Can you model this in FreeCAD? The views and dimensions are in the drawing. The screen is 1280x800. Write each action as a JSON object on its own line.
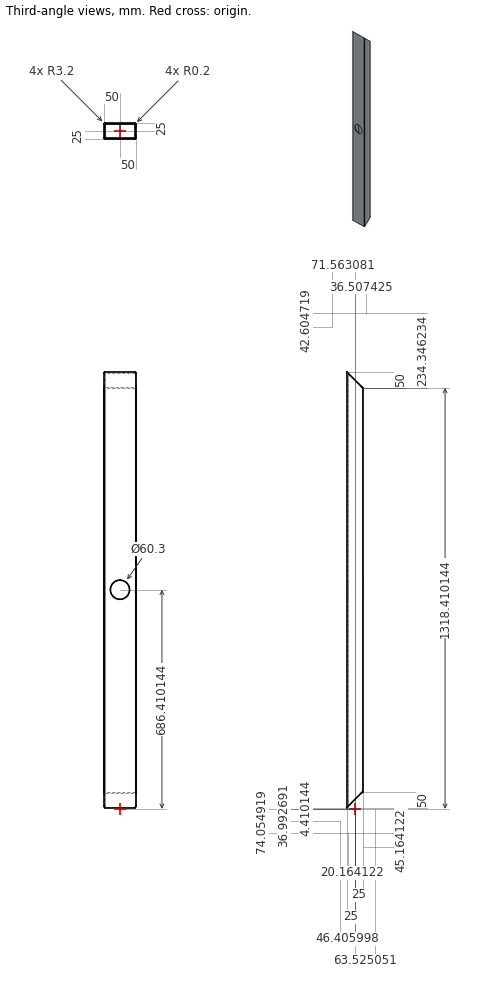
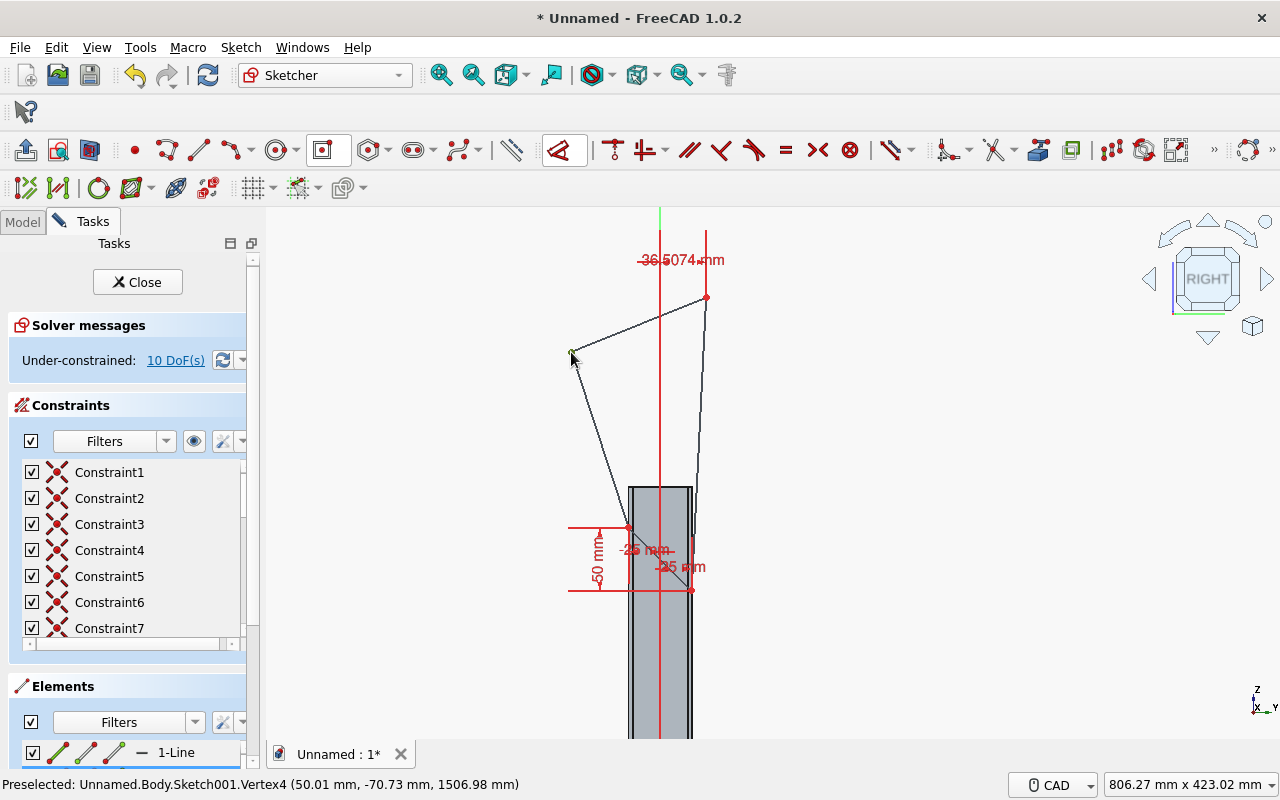
{"action": "key", "text": "l"}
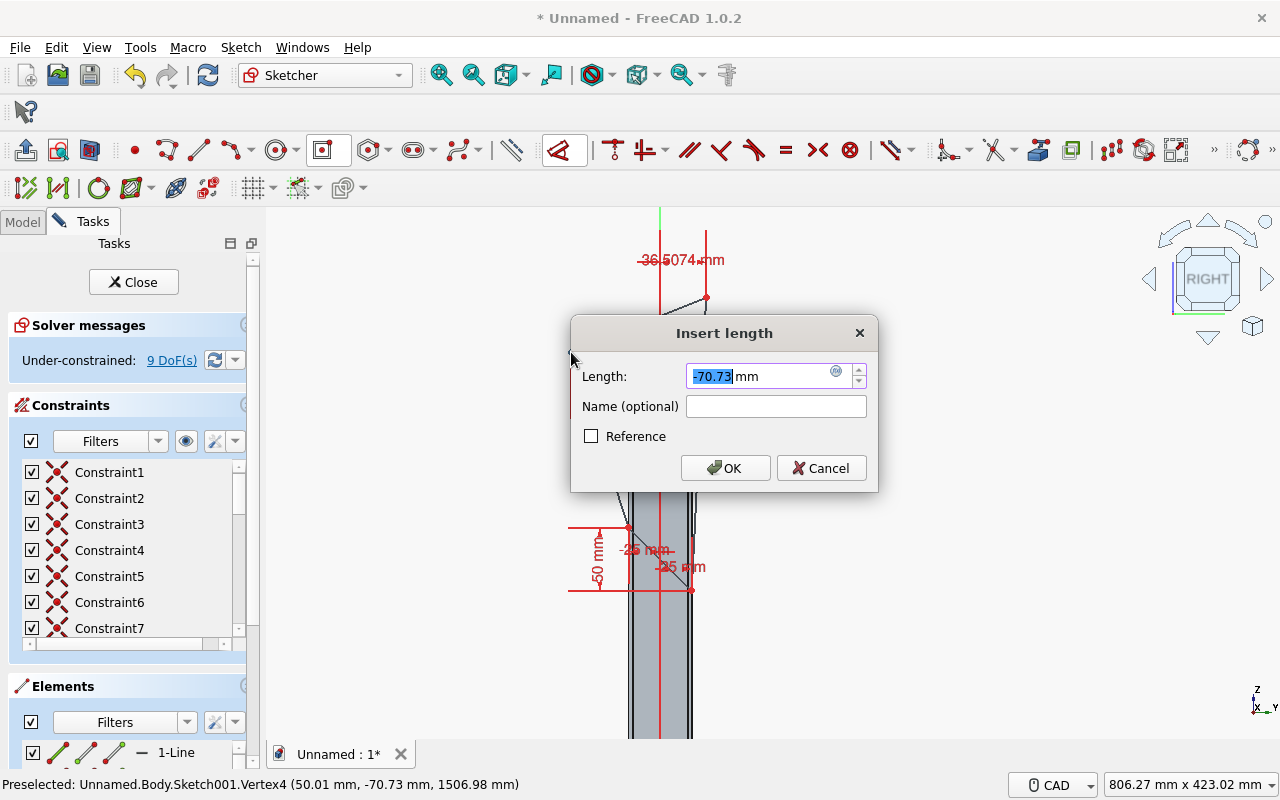
{"action": "type", "text": "-71.563081"}
{"action": "key", "text": "Return"}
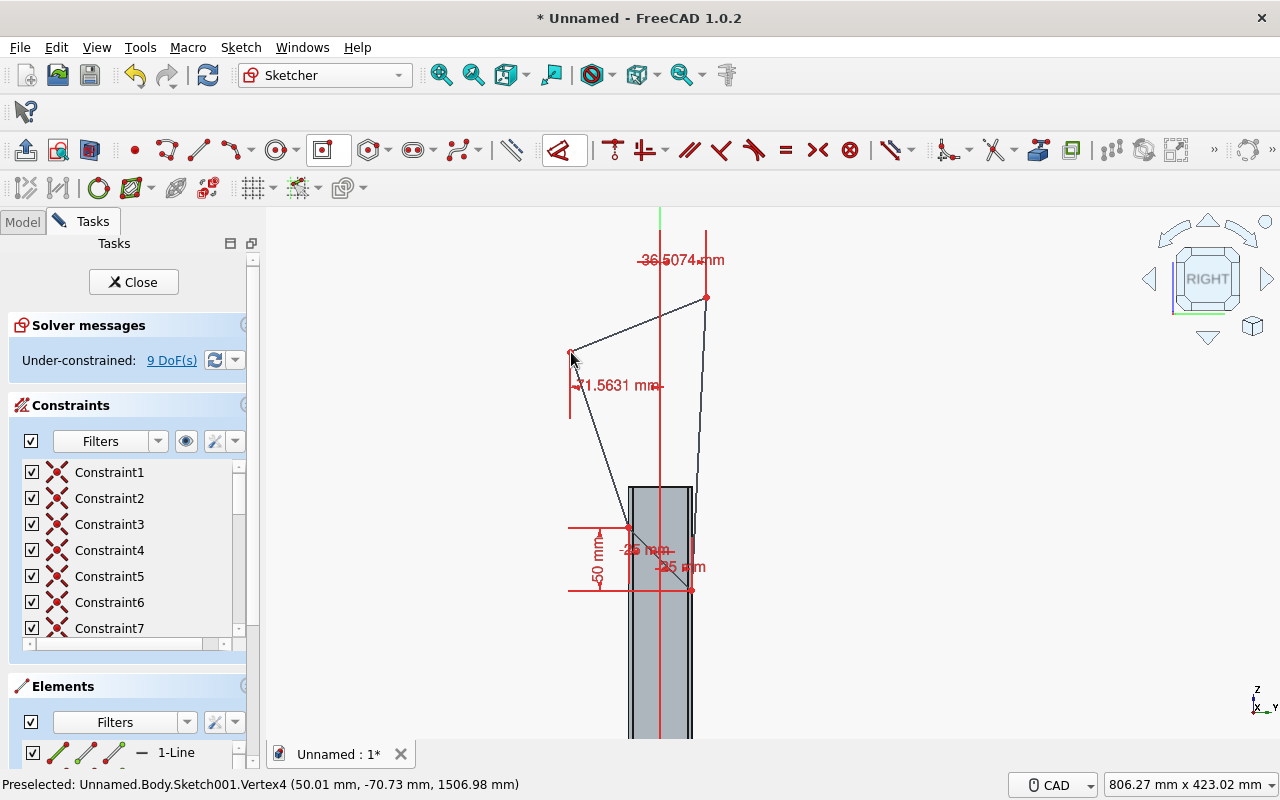
{"action": "scroll", "coordinate": [714, 300], "scroll_direction": "down", "scroll_amount": 9}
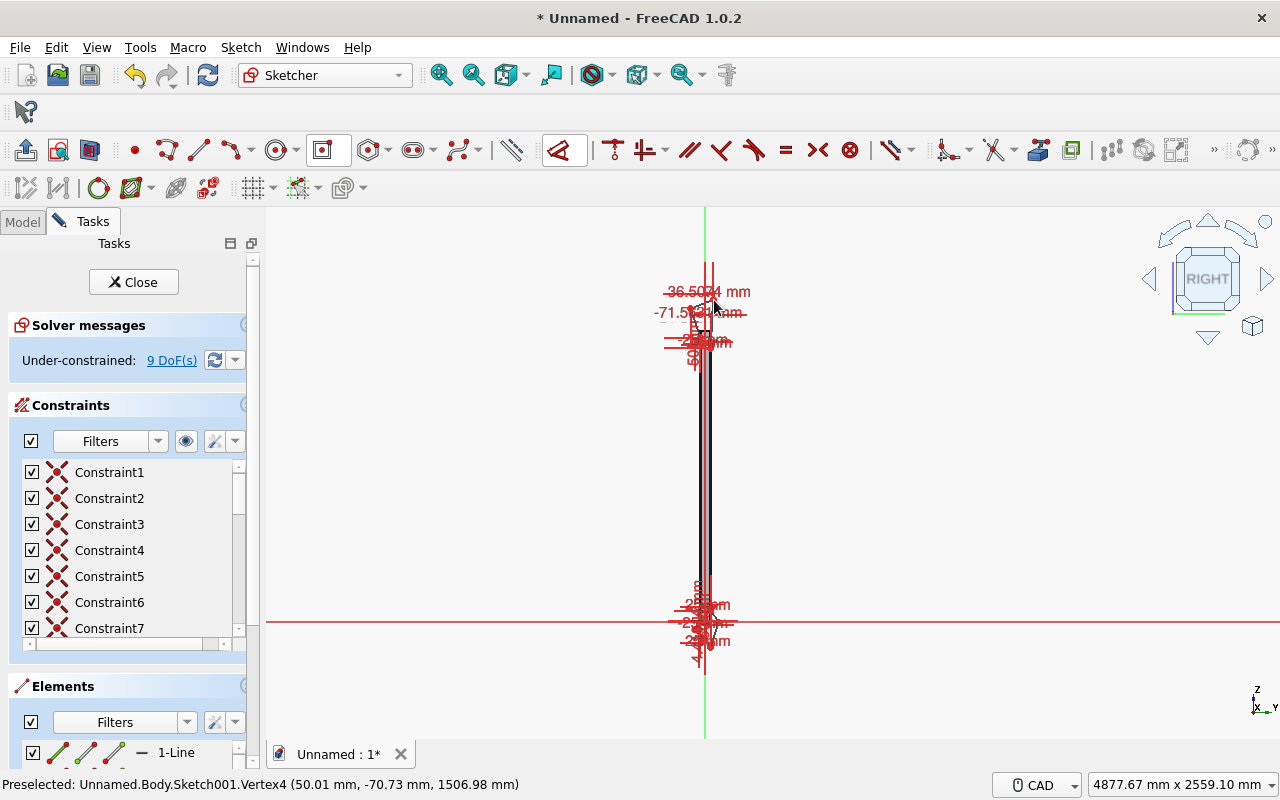
{"action": "scroll", "coordinate": [696, 630], "scroll_direction": "up", "scroll_amount": 8}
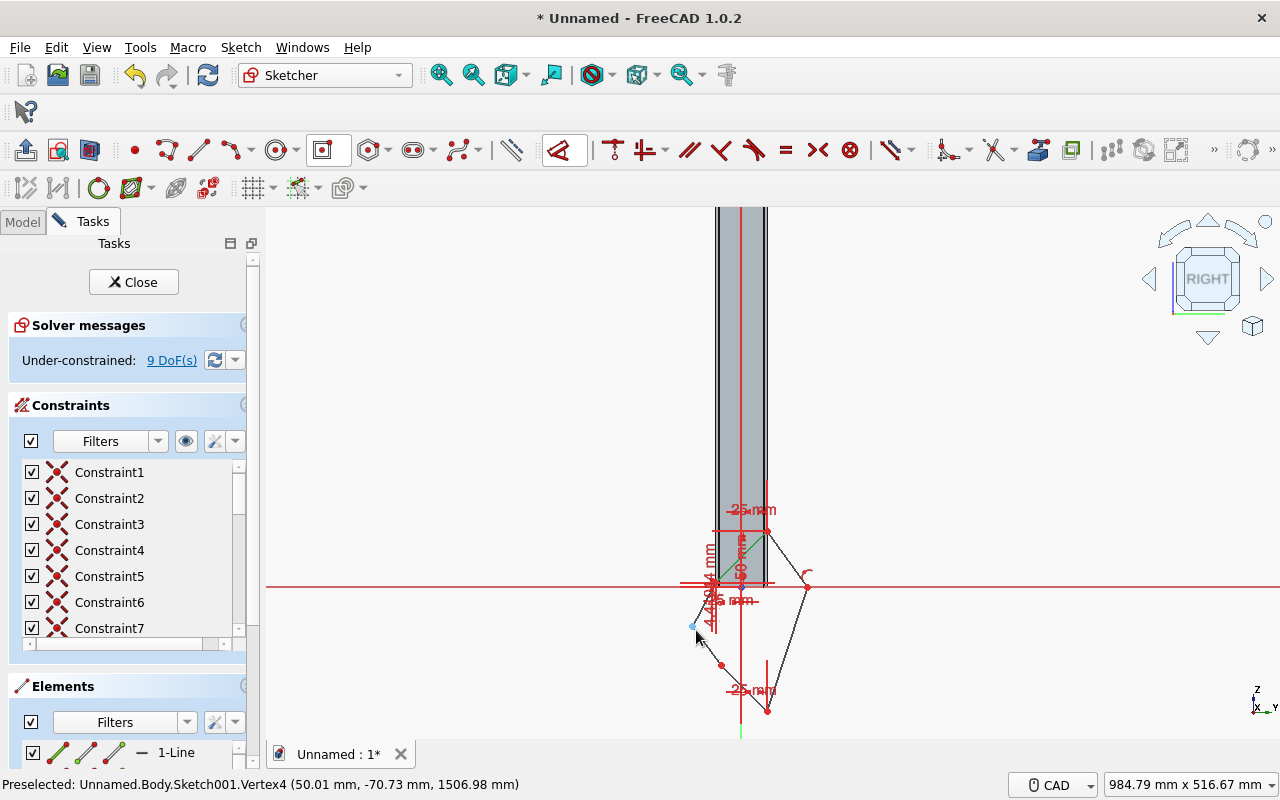
{"action": "left_click", "coordinate": [693, 627]}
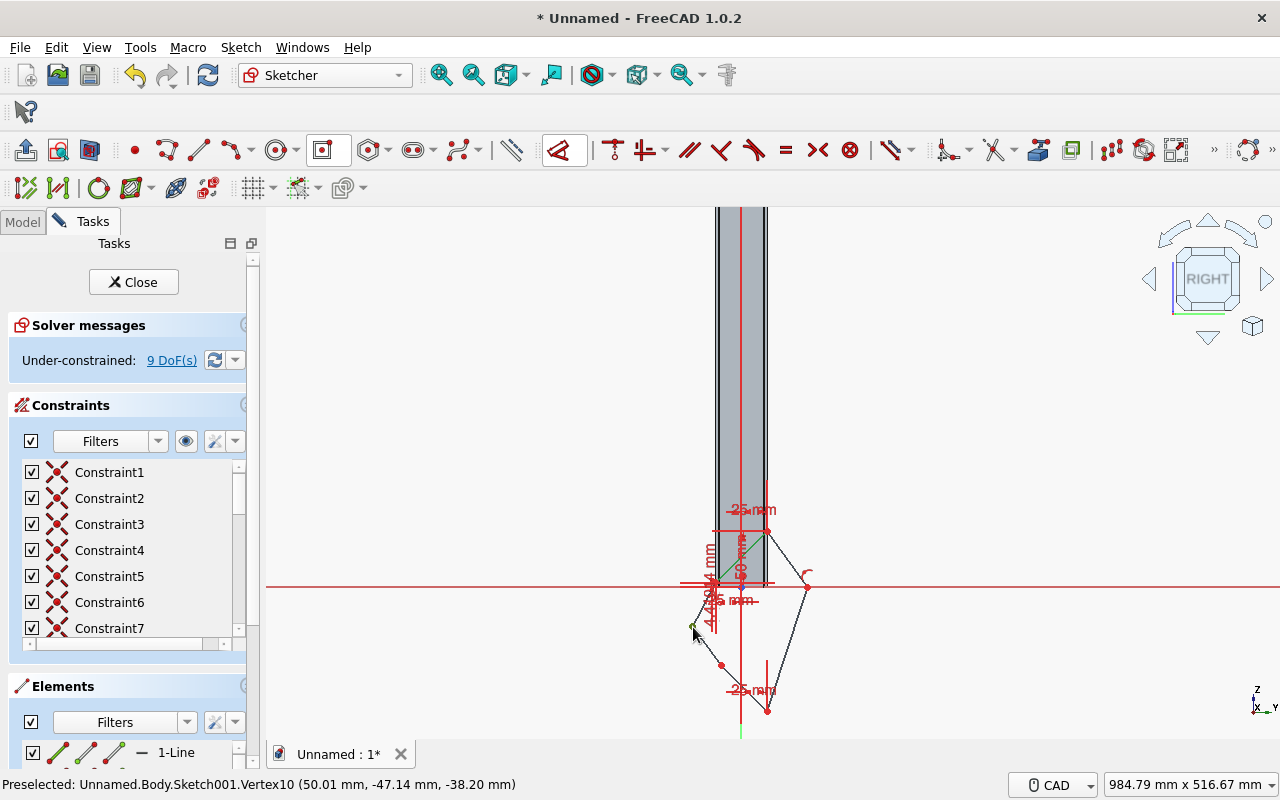
{"action": "key", "text": "l"}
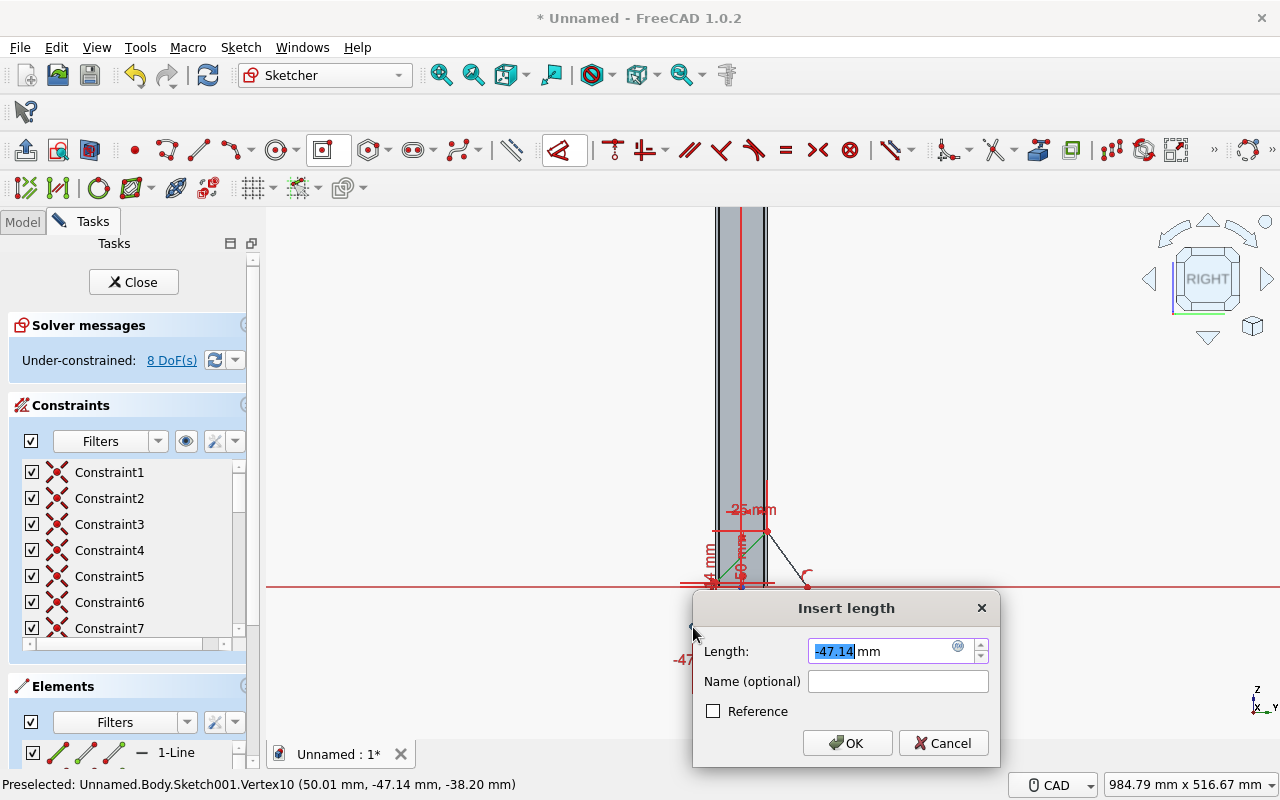
{"action": "type", "text": "-46.405998"}
{"action": "key", "text": "Return"}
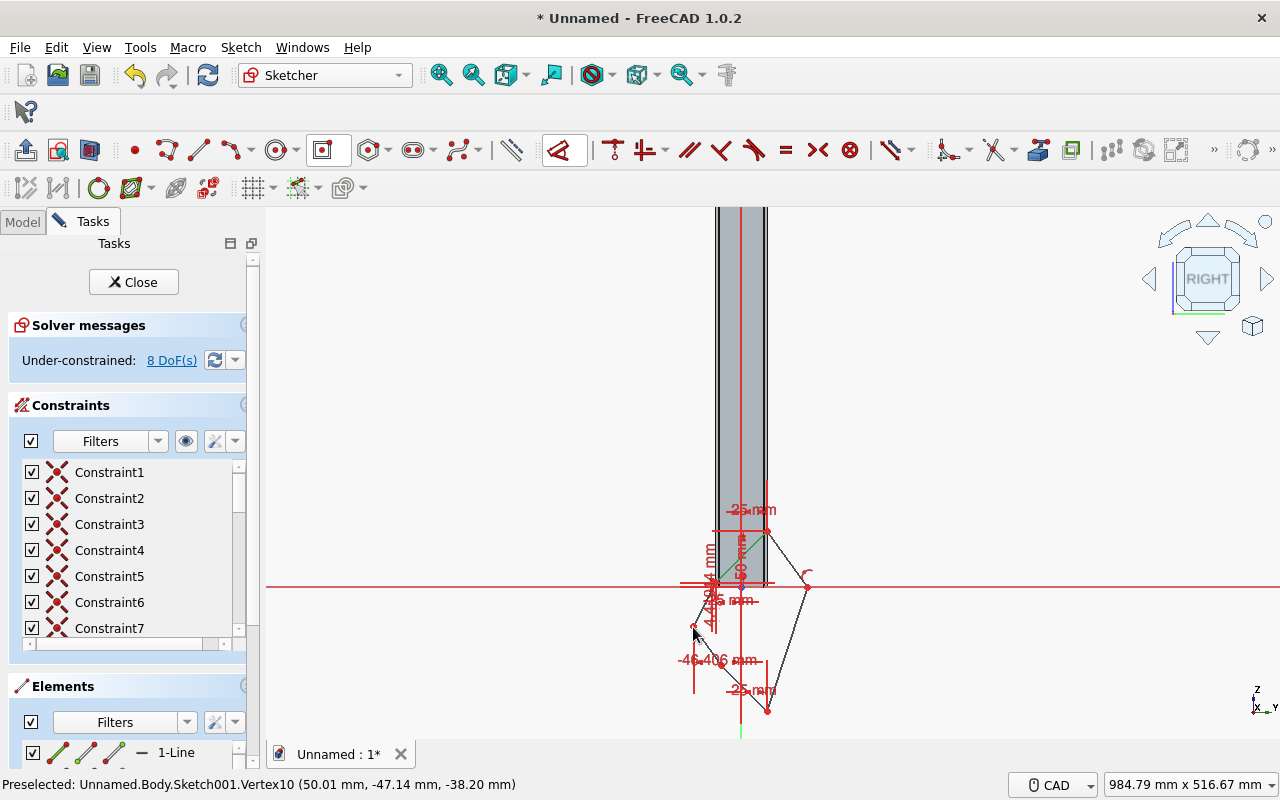
{"action": "left_click", "coordinate": [694, 627]}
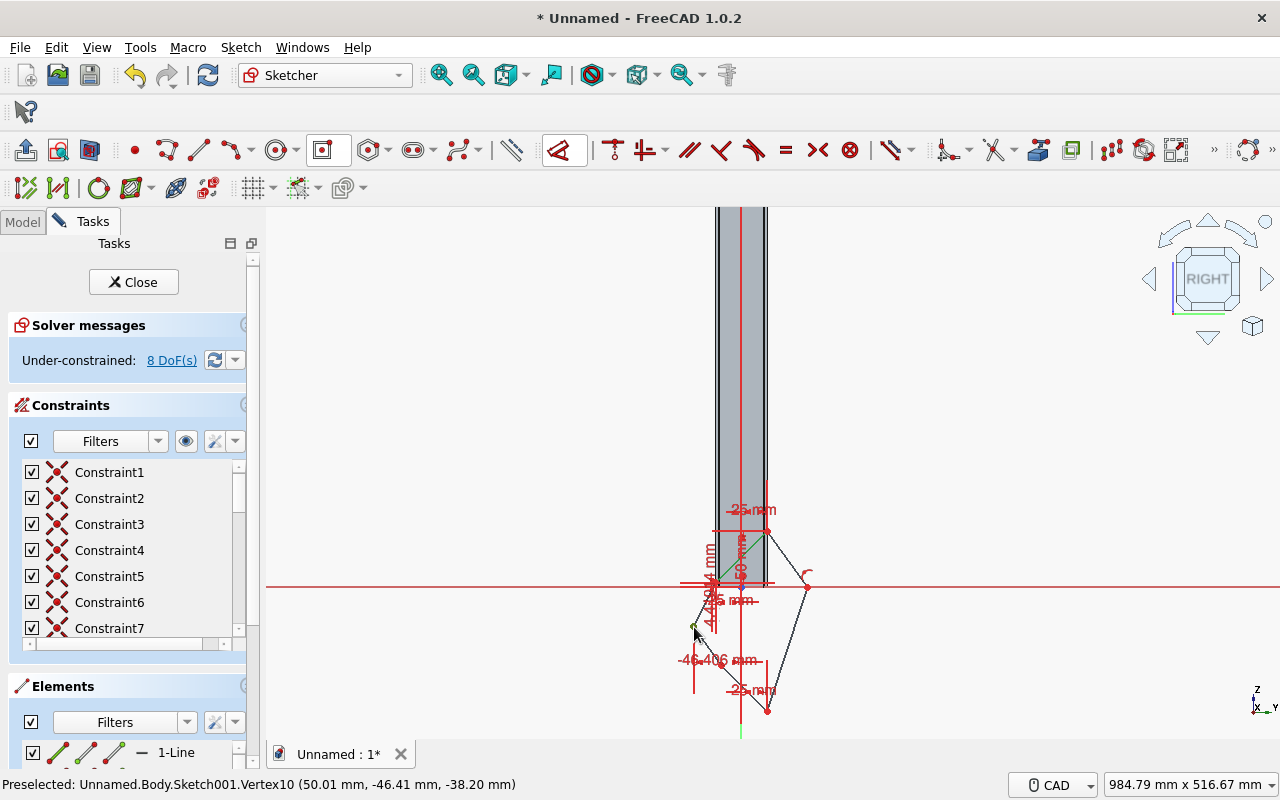
{"action": "key", "text": "i"}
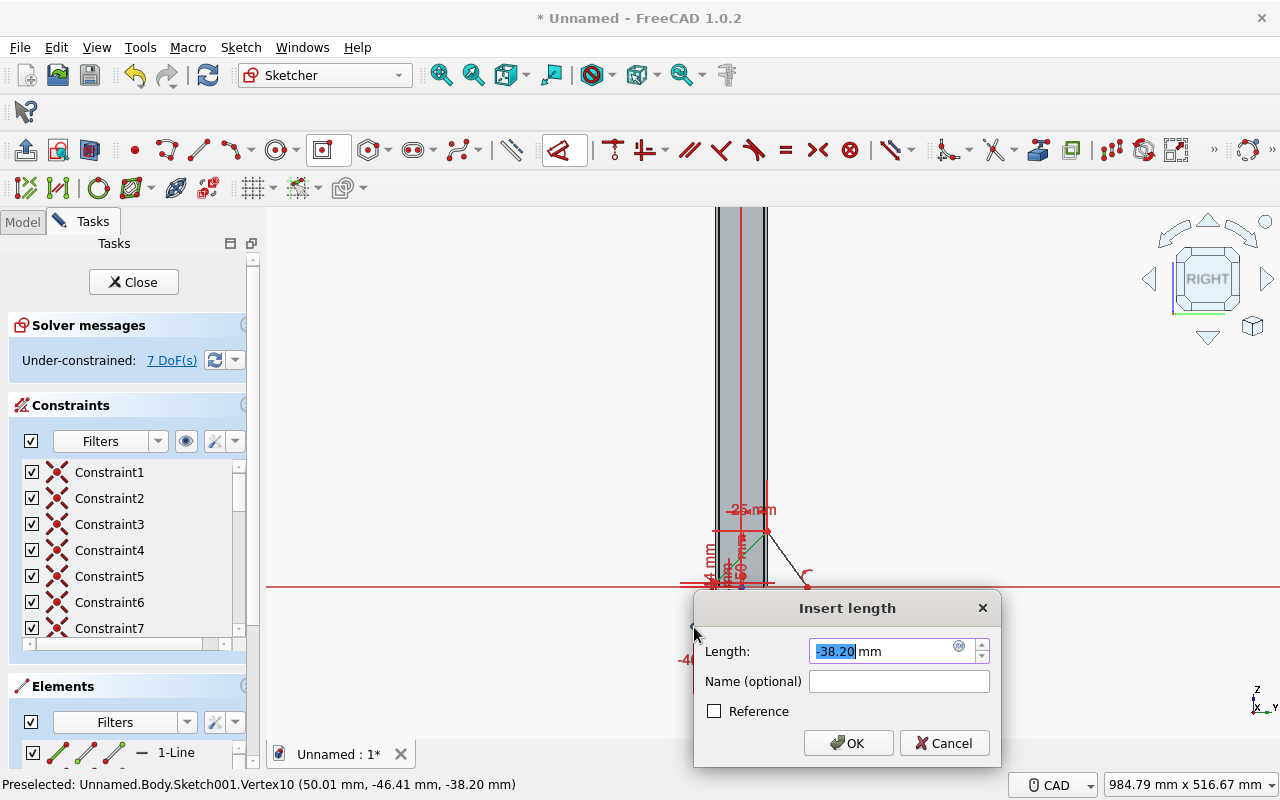
{"action": "type", "text": "-36.992691"}
{"action": "key", "text": "Return"}